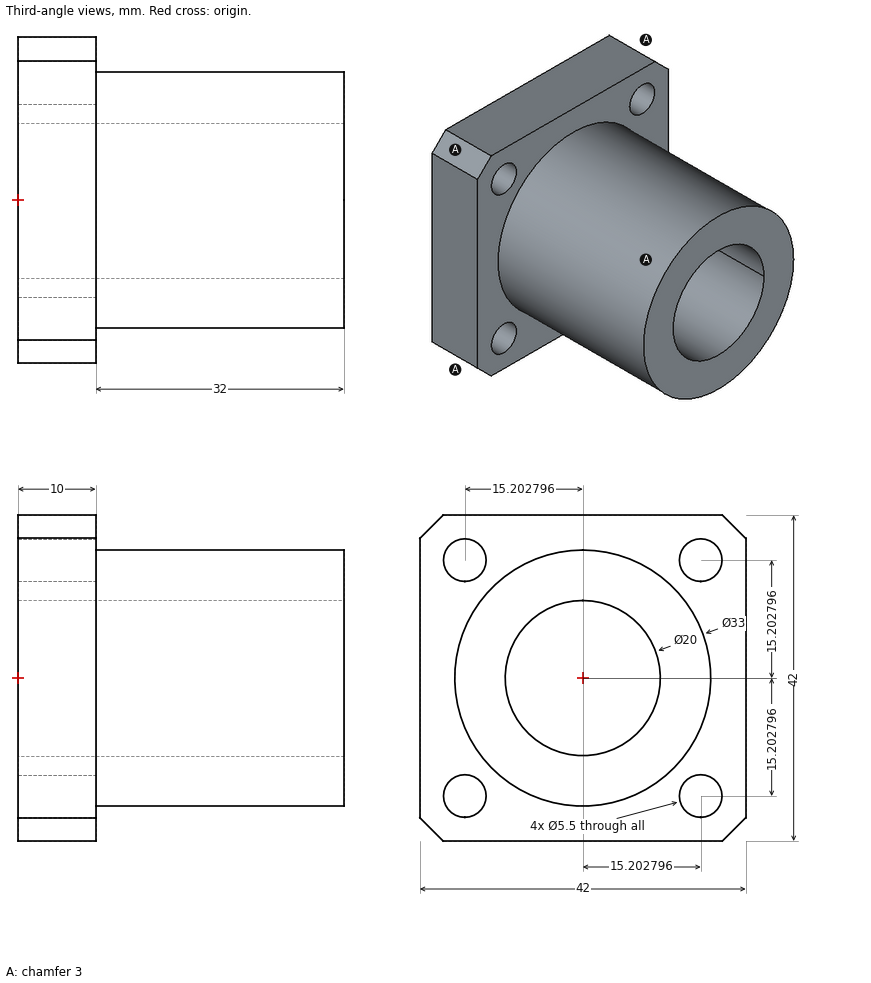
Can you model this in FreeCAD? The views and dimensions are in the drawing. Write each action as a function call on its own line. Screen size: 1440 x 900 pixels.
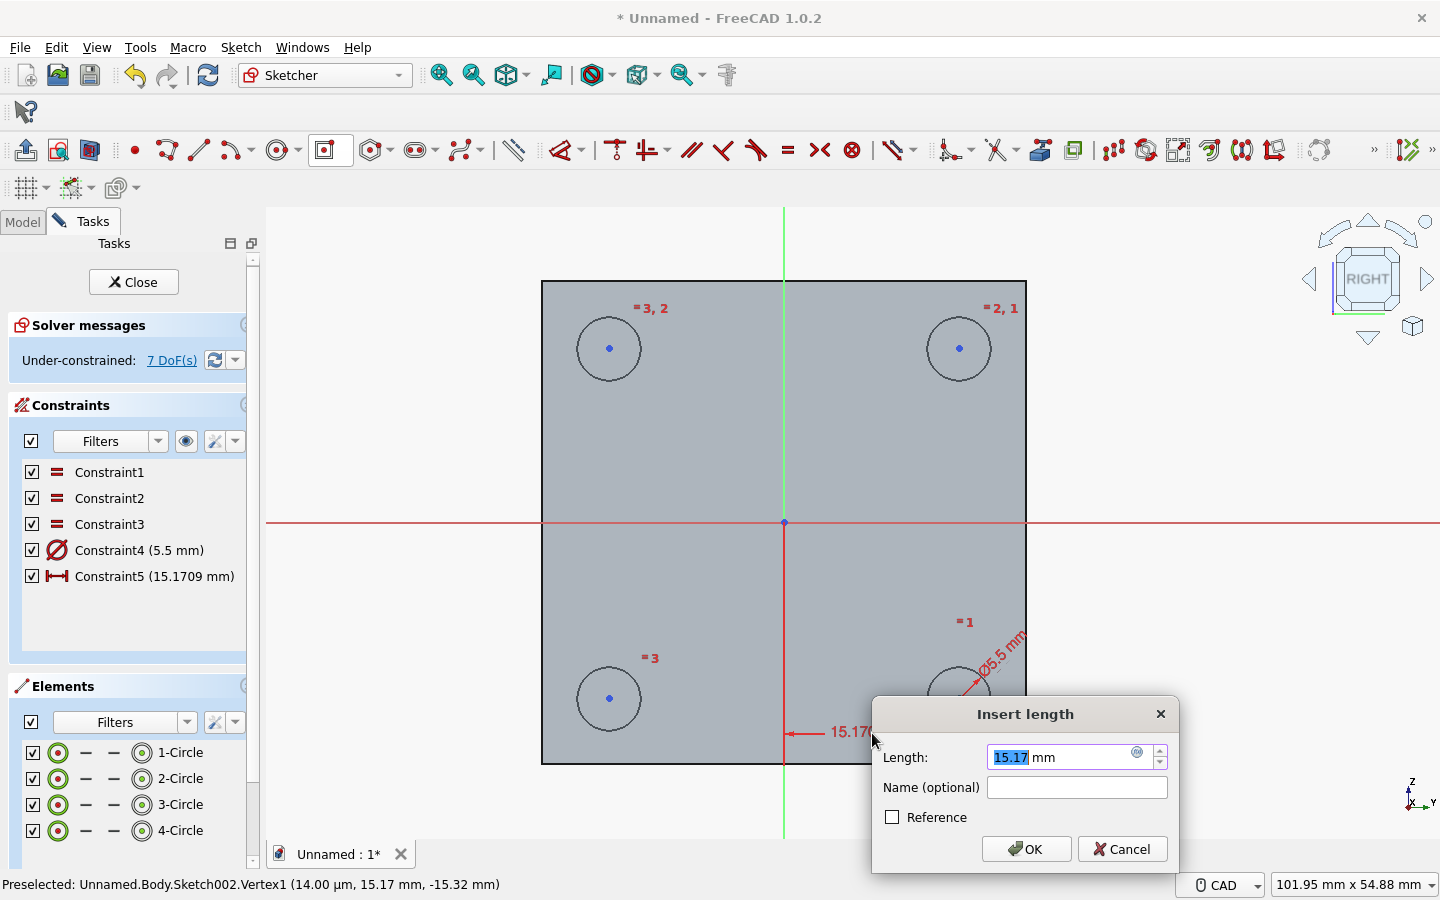
text(15.202796)
key(Return)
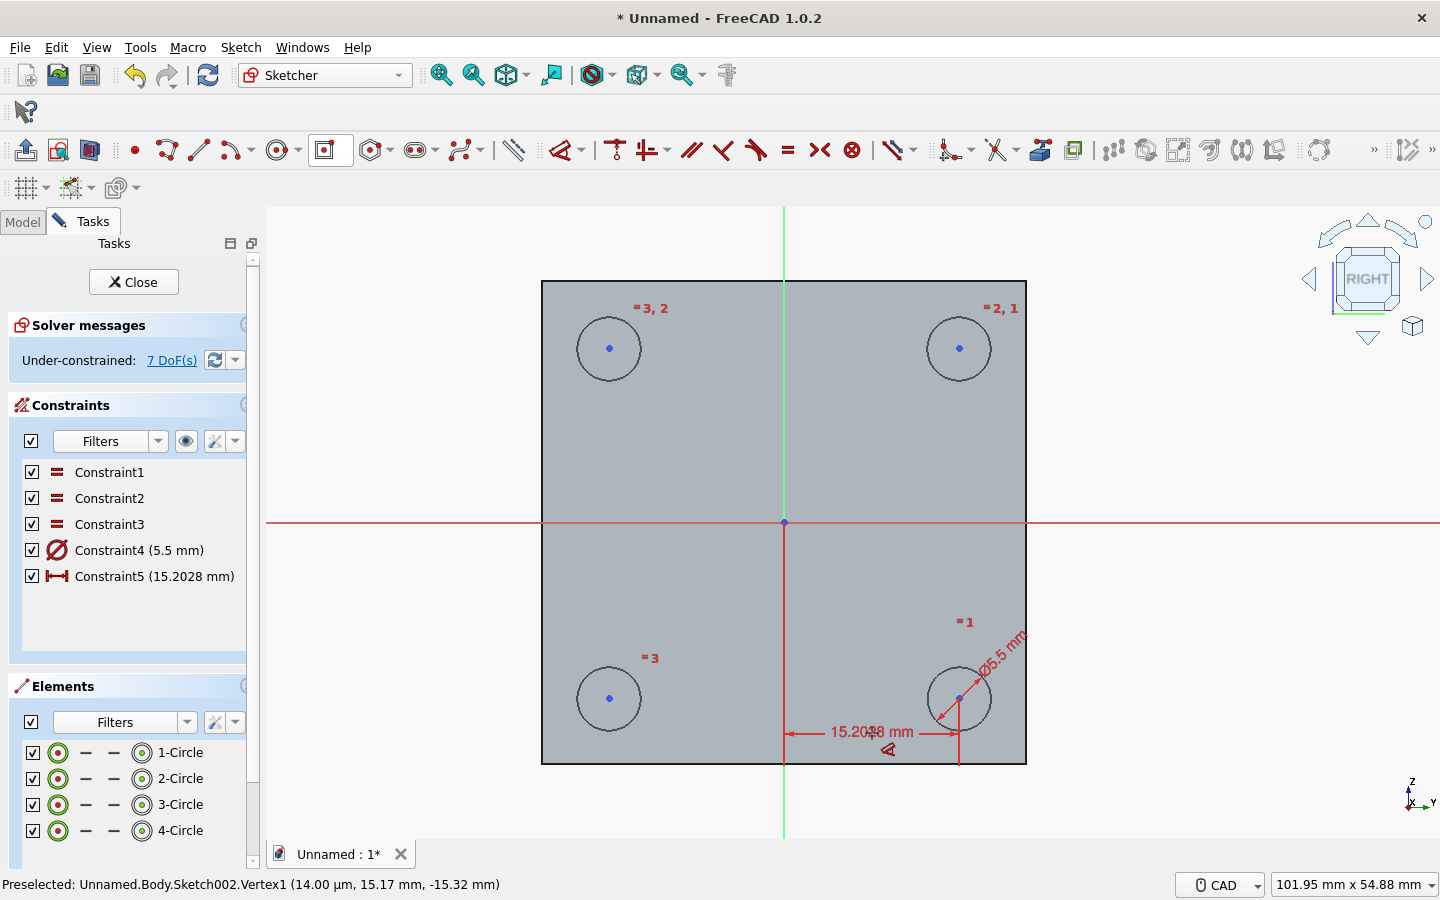
click(959, 699)
click(993, 611)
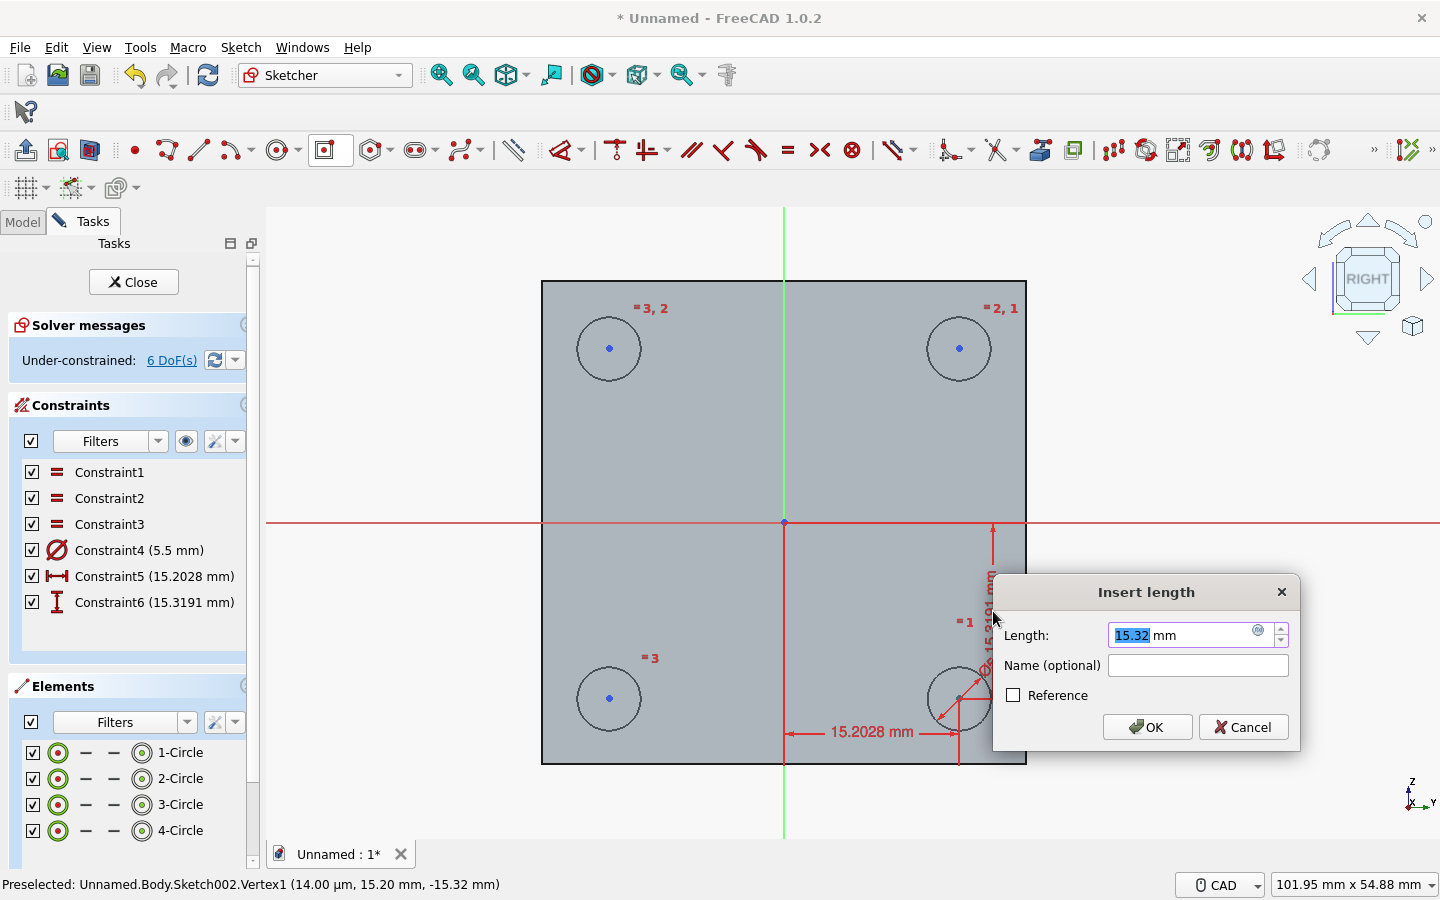
text(15.202796)
key(Return)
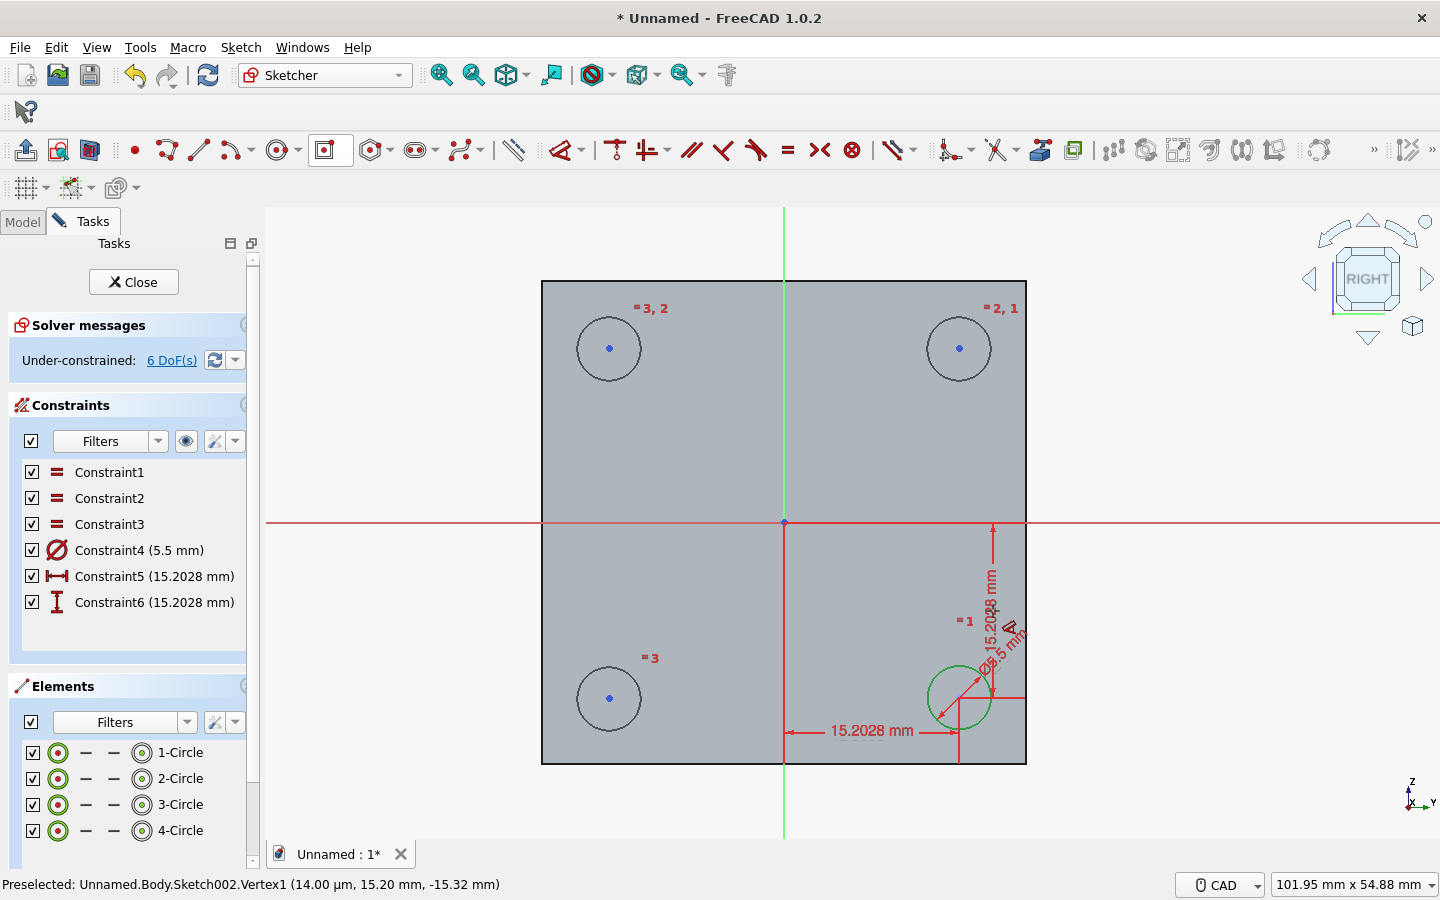
click(959, 349)
click(872, 315)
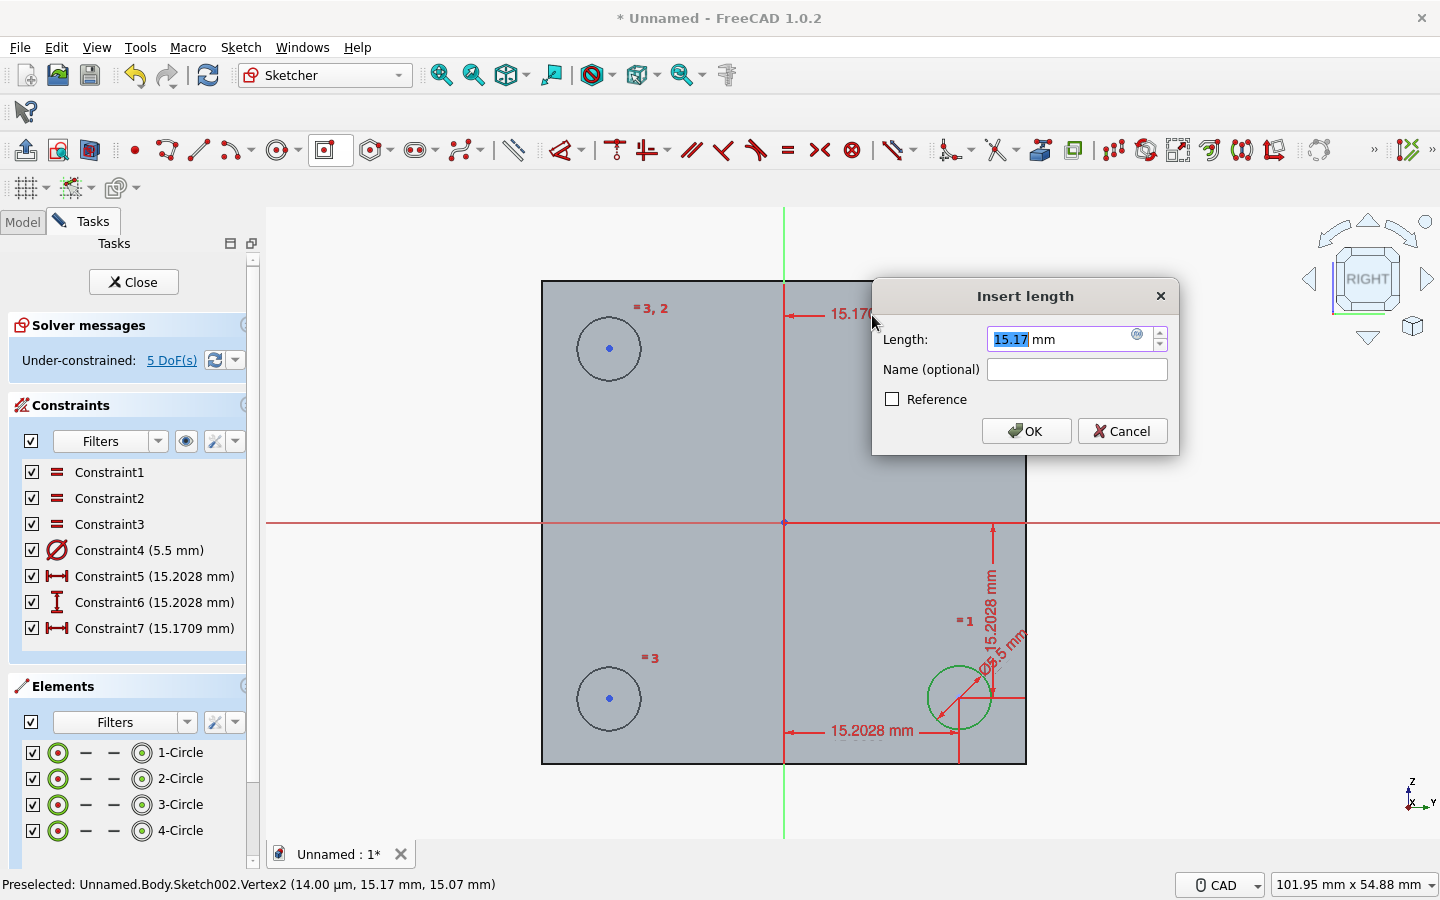
text(15.202796)
key(Return)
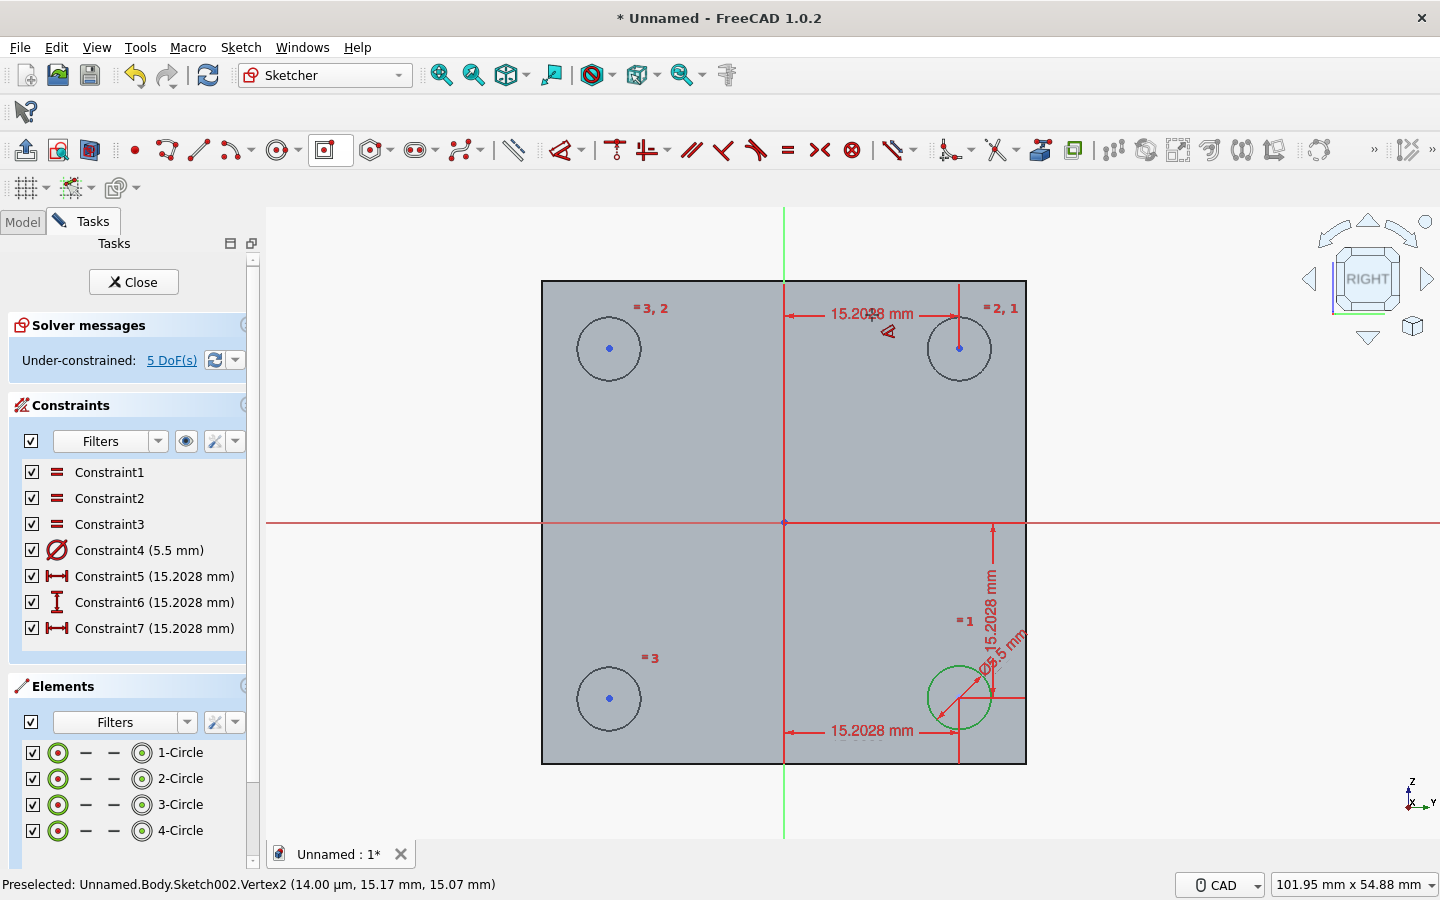
click(959, 349)
click(993, 436)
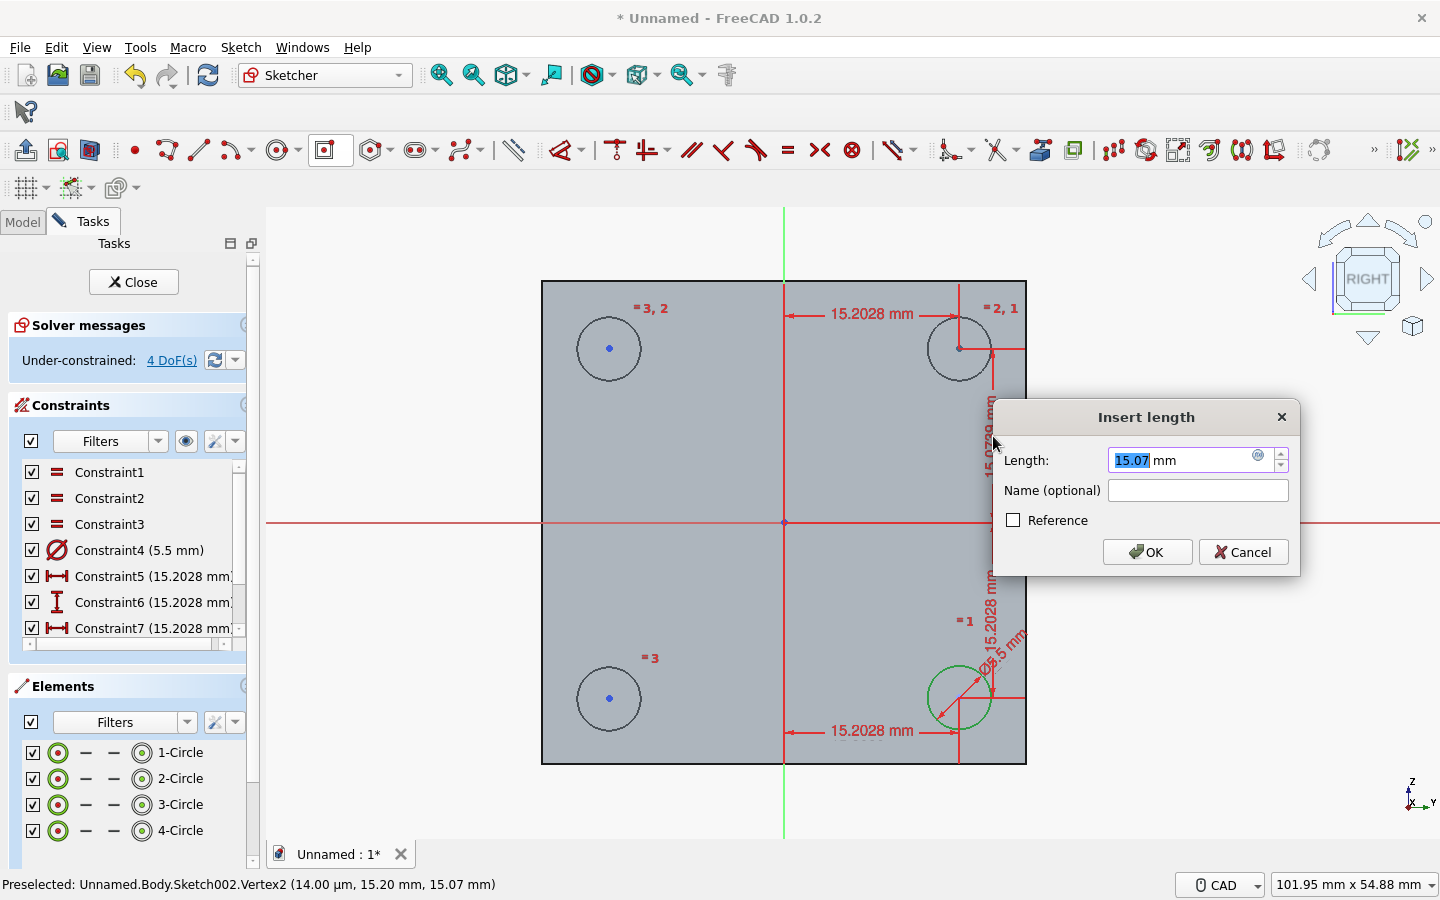
text(15.202796)
key(Return)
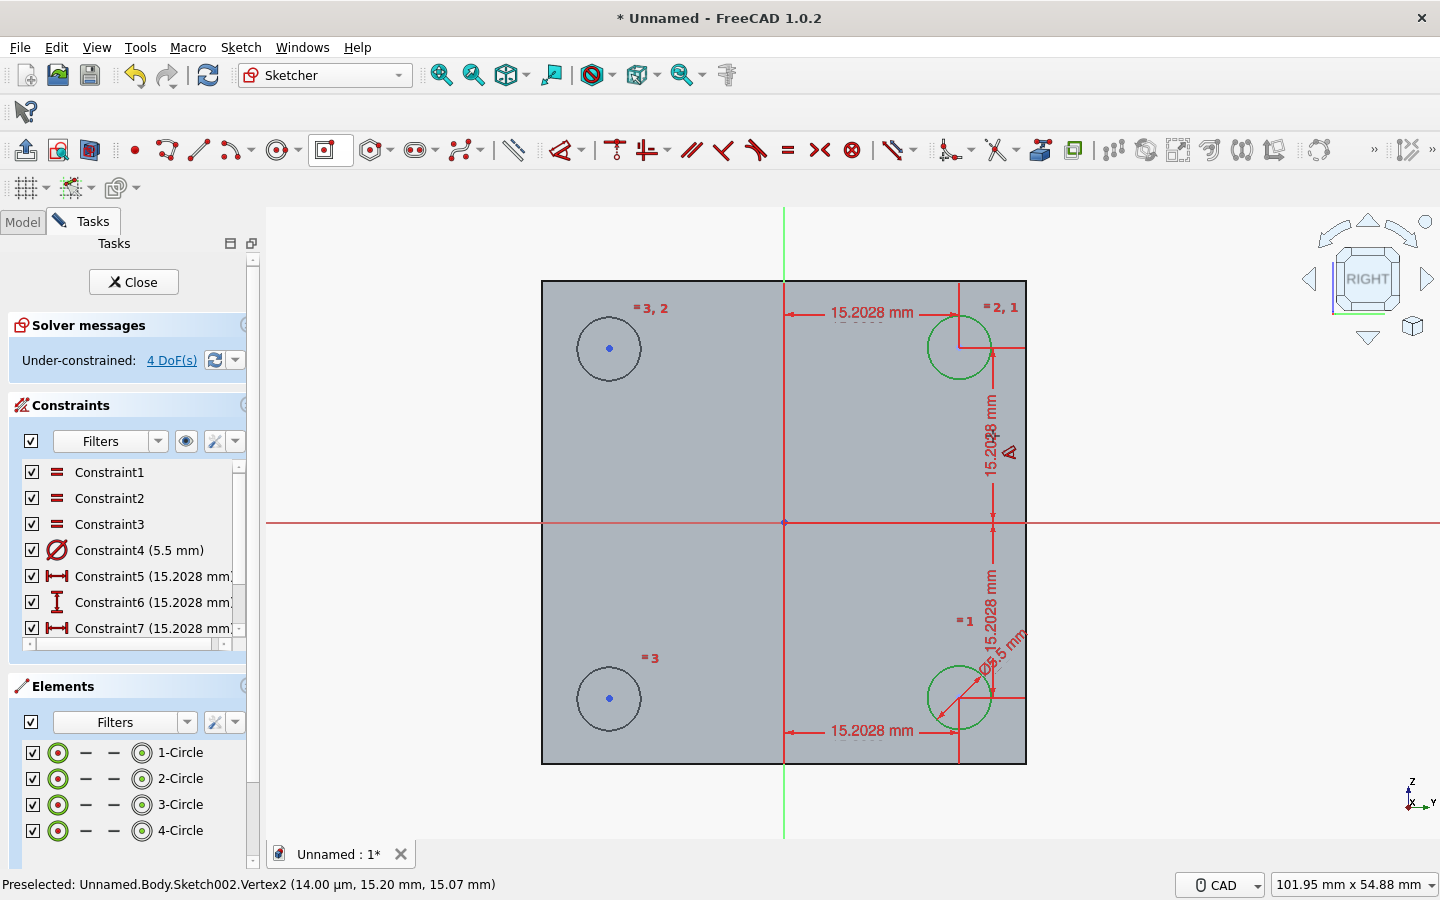
click(609, 349)
click(697, 315)